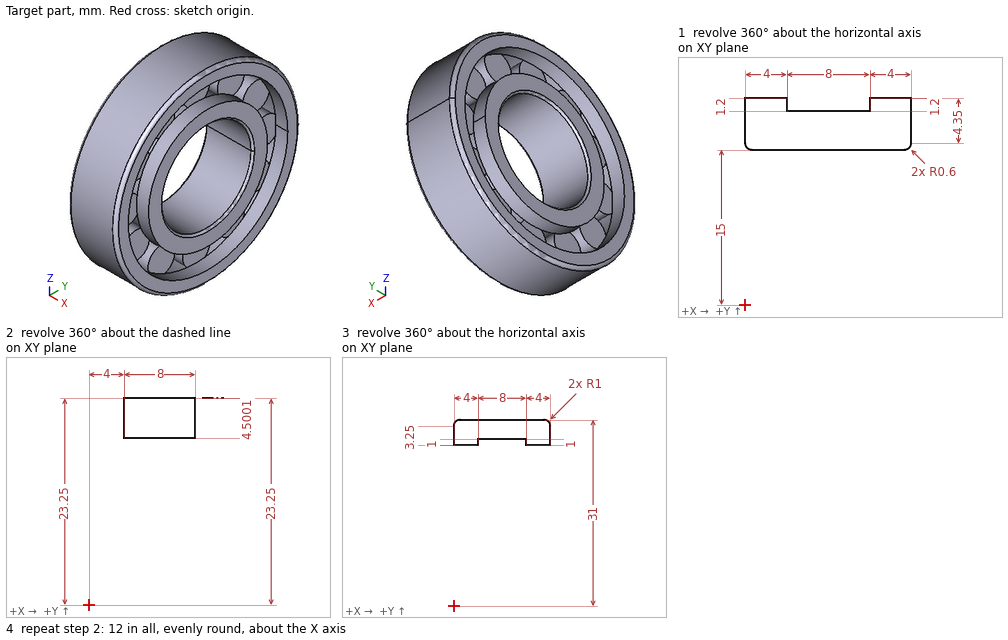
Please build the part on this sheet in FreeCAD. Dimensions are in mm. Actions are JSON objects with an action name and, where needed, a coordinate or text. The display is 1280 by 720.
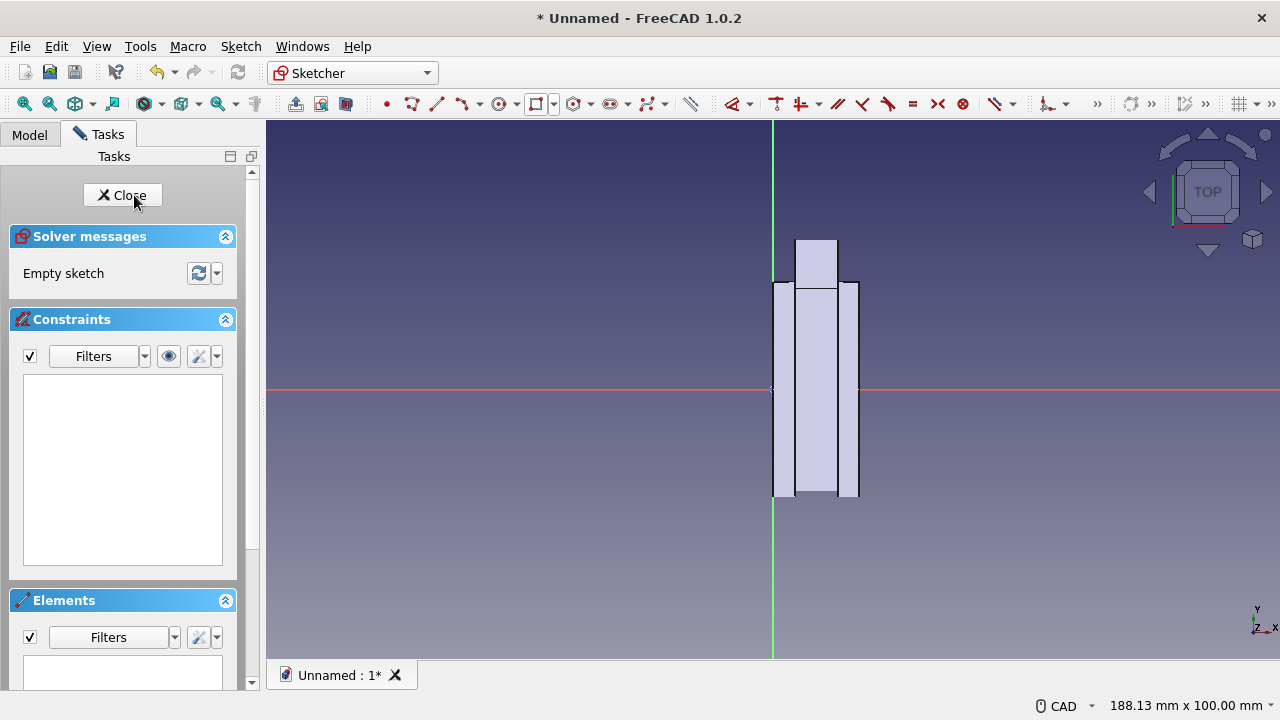
{"action": "left_click", "coordinate": [346, 104]}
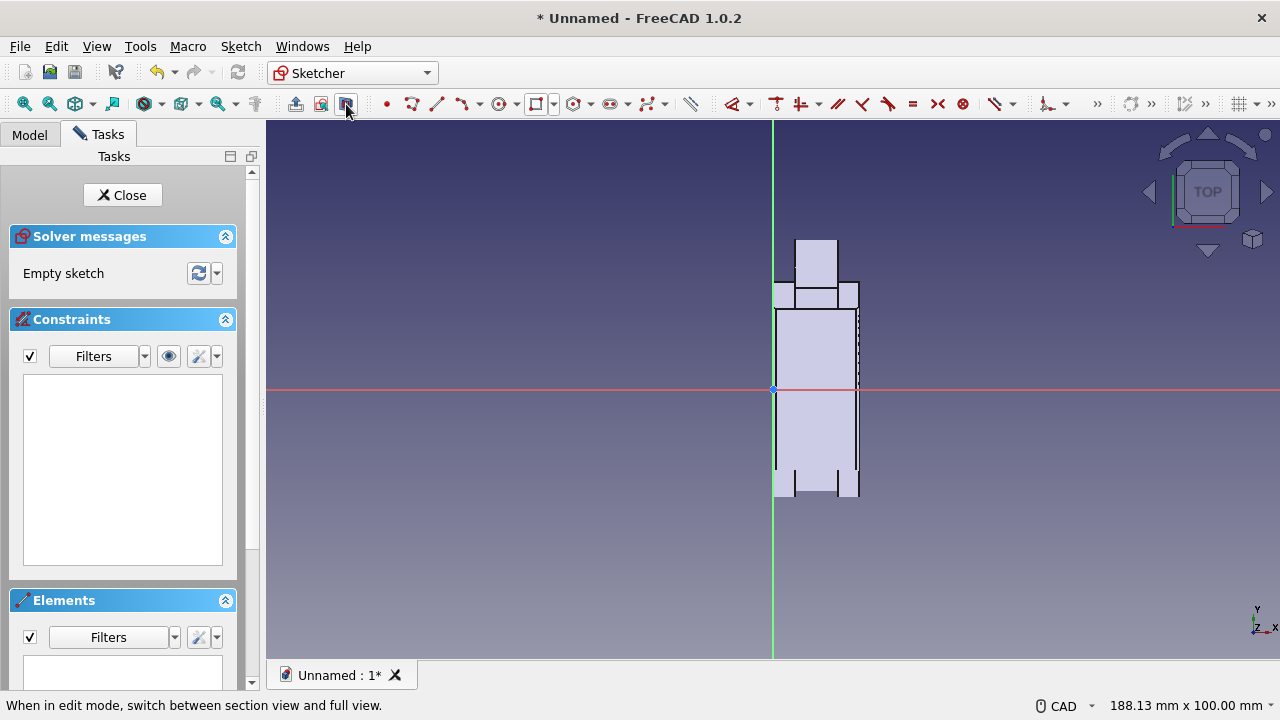
{"action": "scroll", "coordinate": [907, 238], "scroll_direction": "up", "scroll_amount": 4}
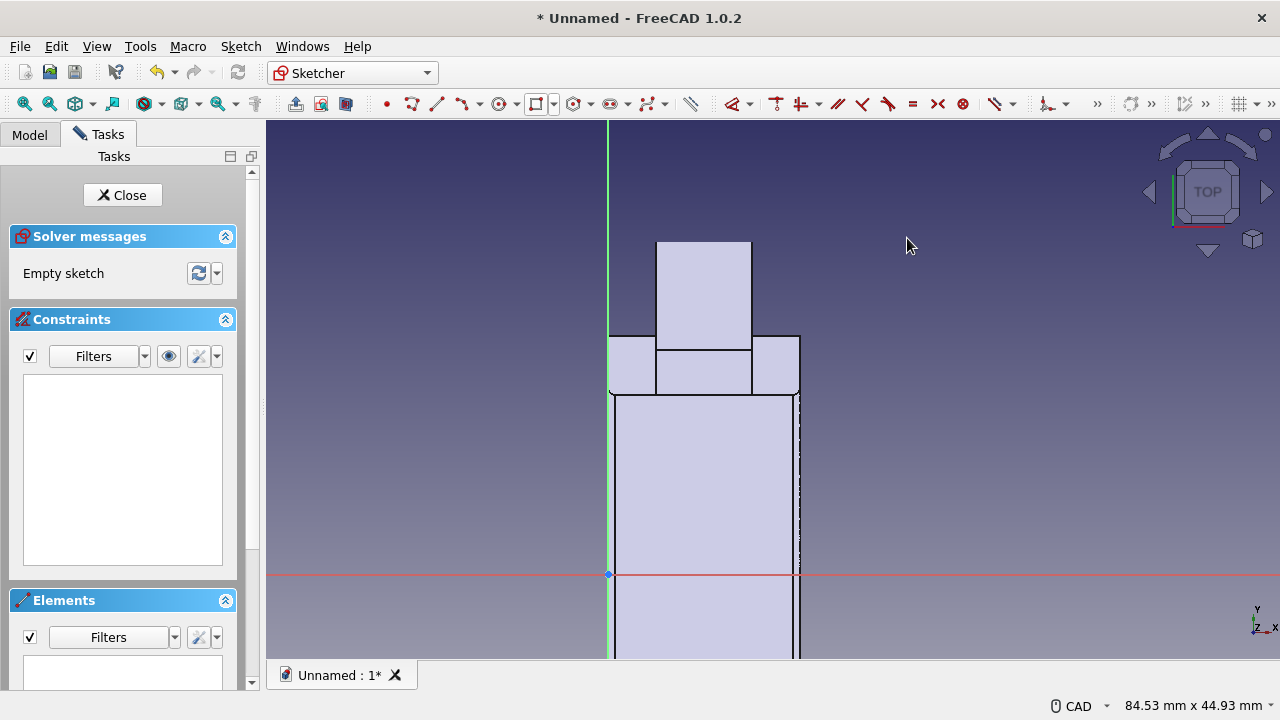
{"action": "left_click", "coordinate": [437, 104]}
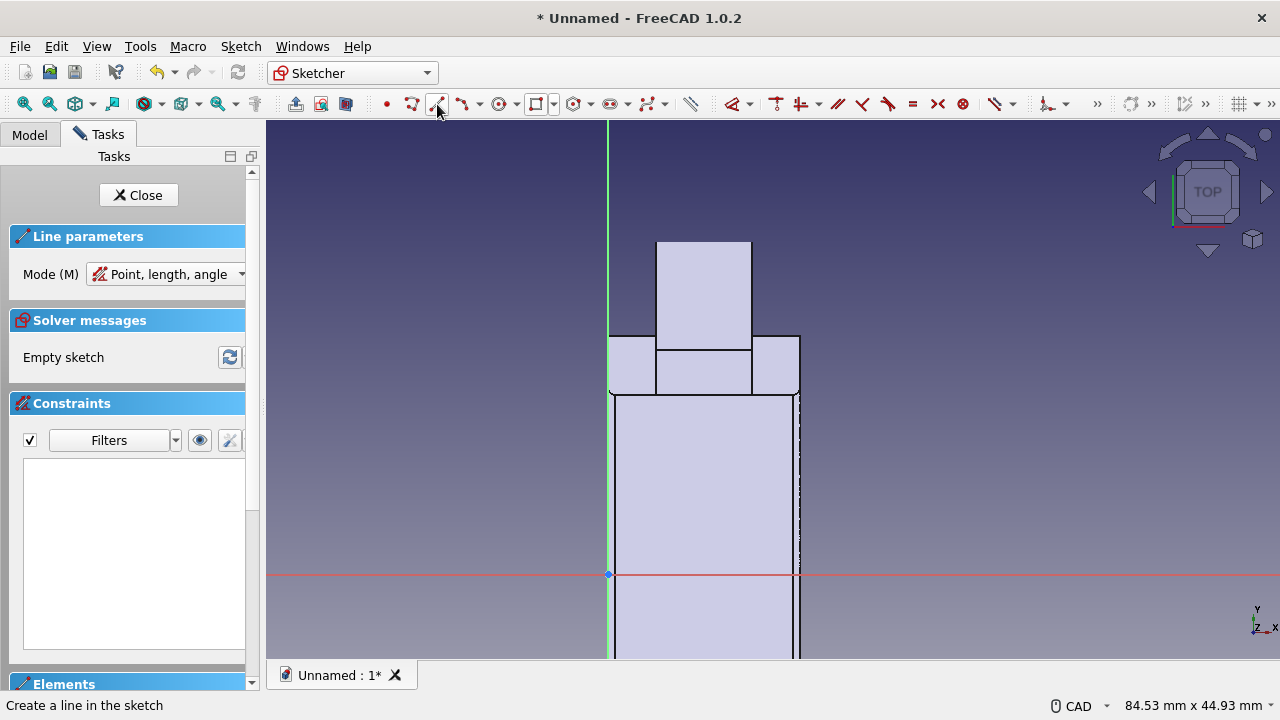
{"action": "left_click", "coordinate": [788, 203]}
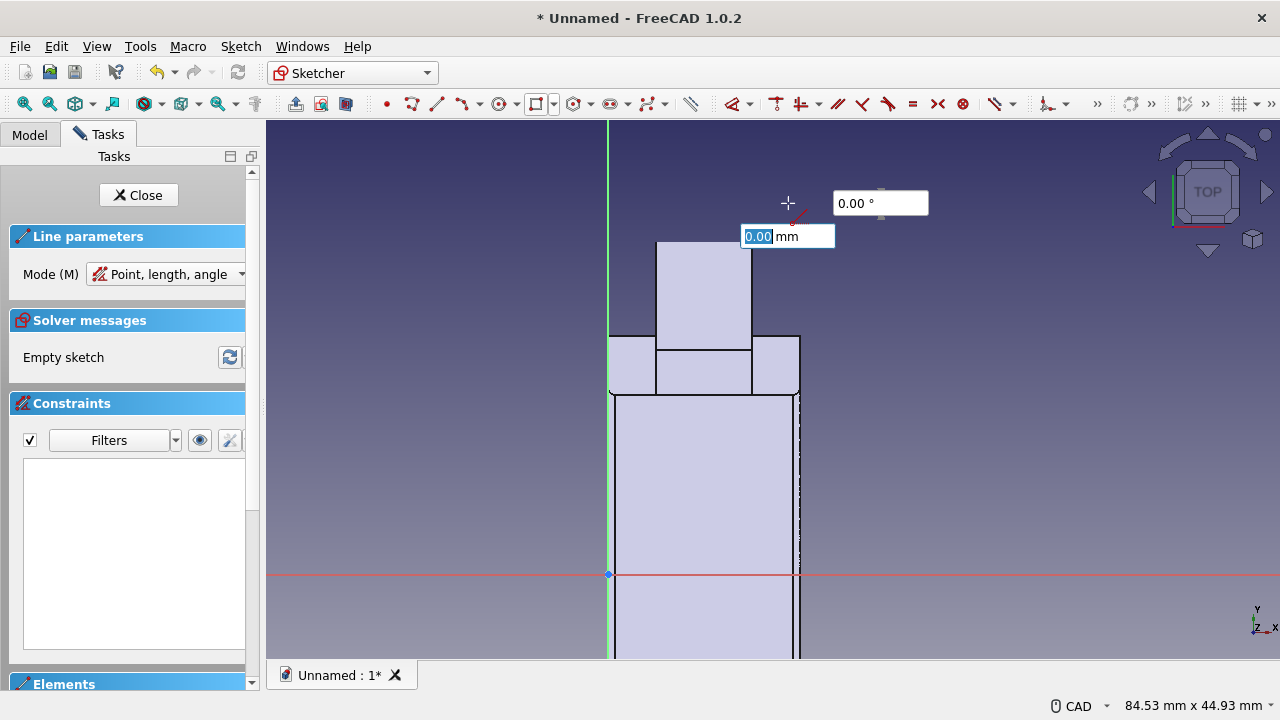
{"action": "scroll", "coordinate": [620, 203], "scroll_direction": "up", "scroll_amount": 2}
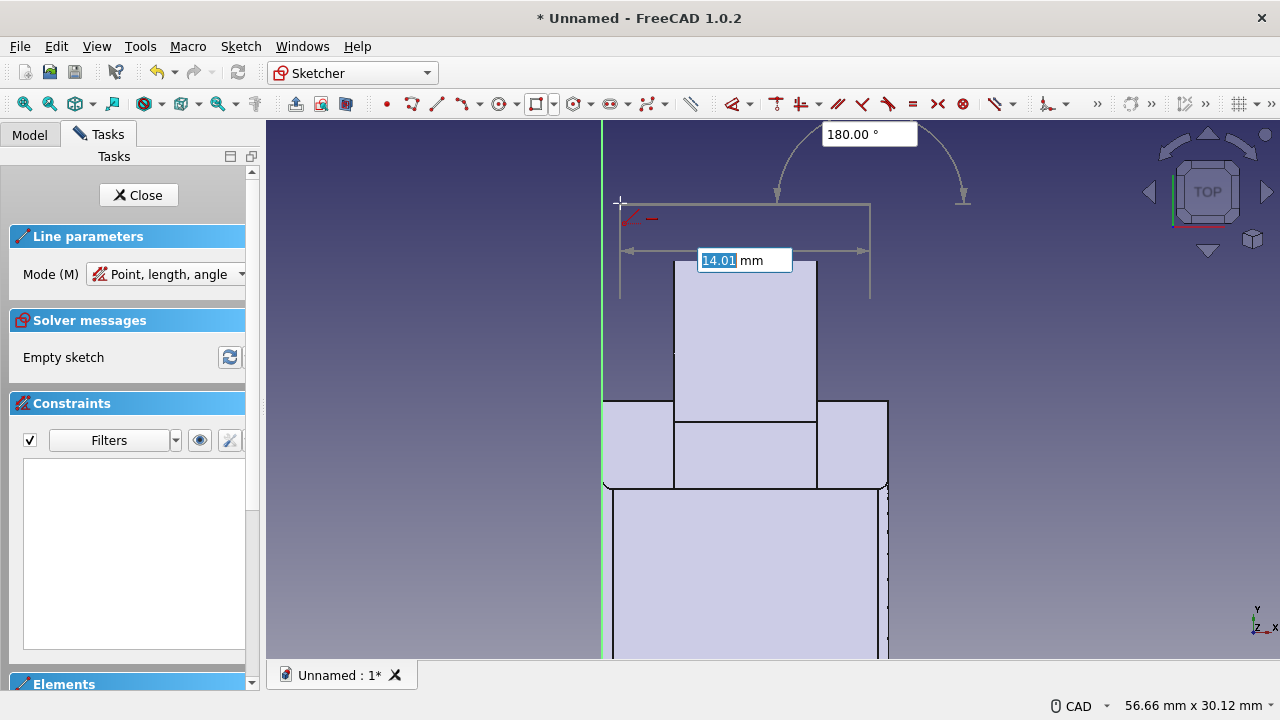
{"action": "left_click", "coordinate": [620, 203]}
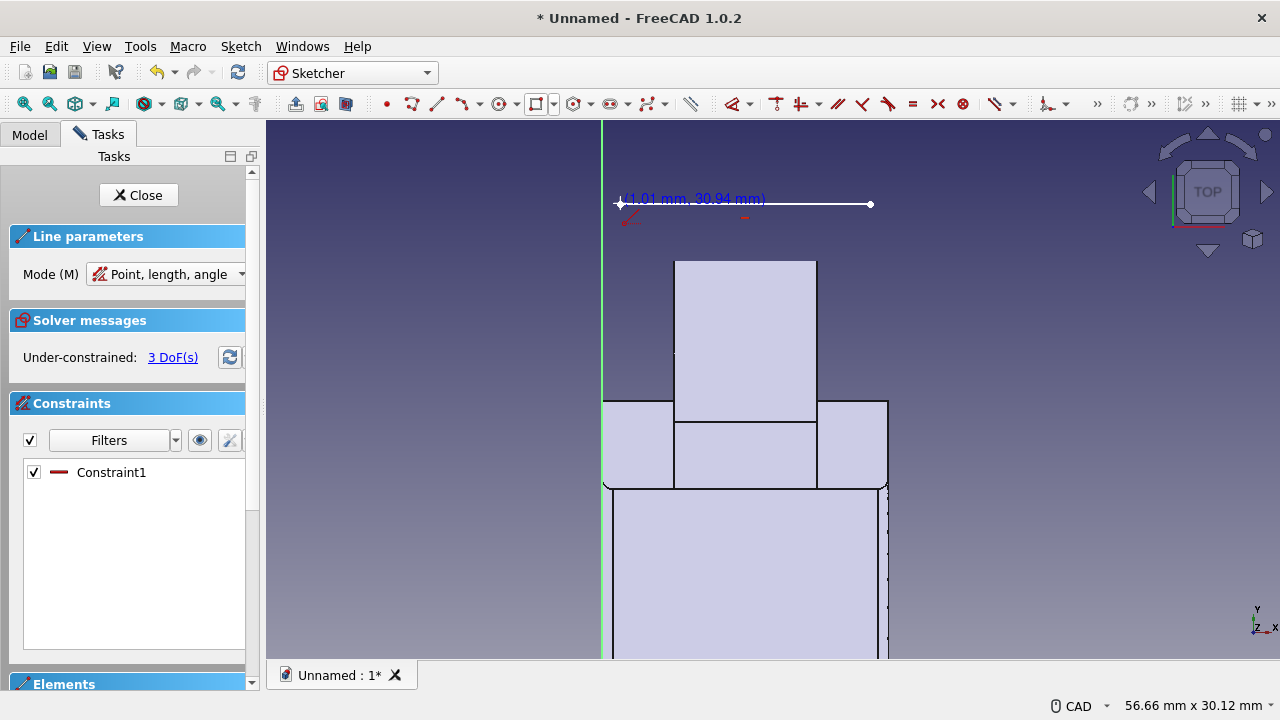
{"action": "left_click", "coordinate": [412, 104]}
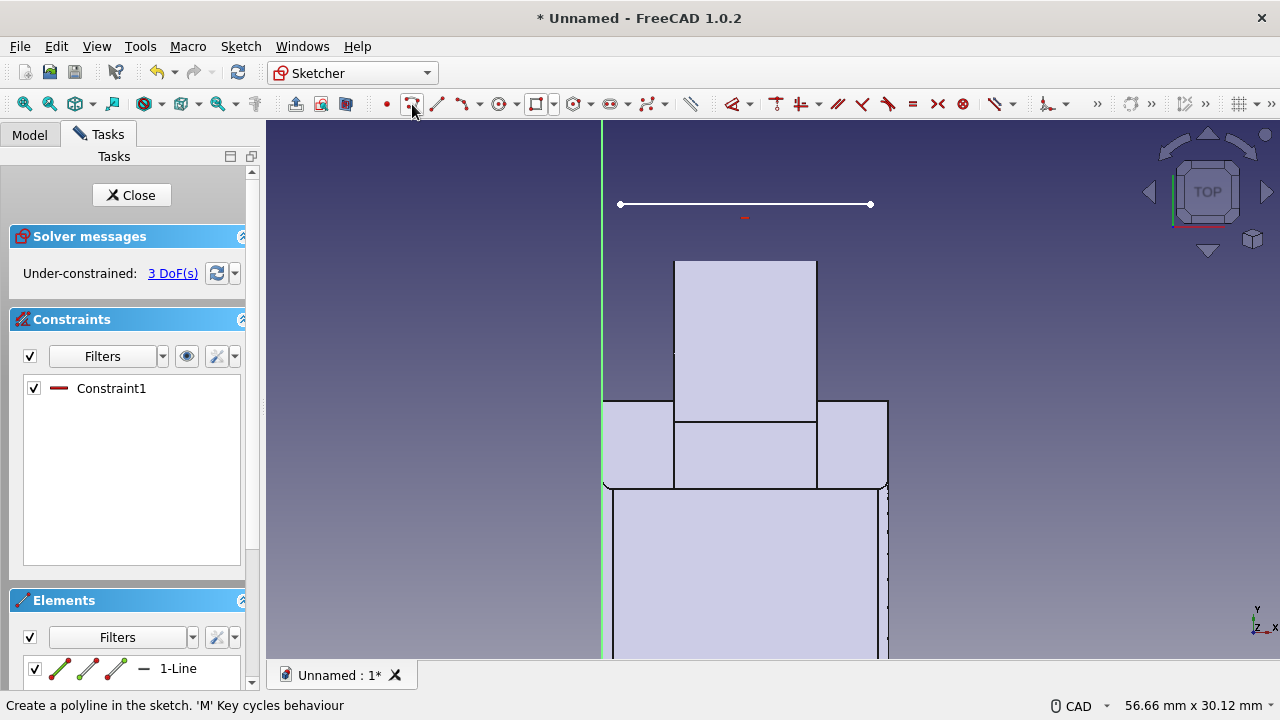
{"action": "left_click", "coordinate": [602, 221]}
{"action": "left_click", "coordinate": [611, 279]}
{"action": "left_click", "coordinate": [674, 279]}
{"action": "left_click", "coordinate": [674, 261]}
{"action": "left_click", "coordinate": [817, 261]}
{"action": "left_click", "coordinate": [817, 279]}
{"action": "left_click", "coordinate": [888, 279]}
{"action": "left_click", "coordinate": [888, 221]}
{"action": "right_click", "coordinate": [888, 221]}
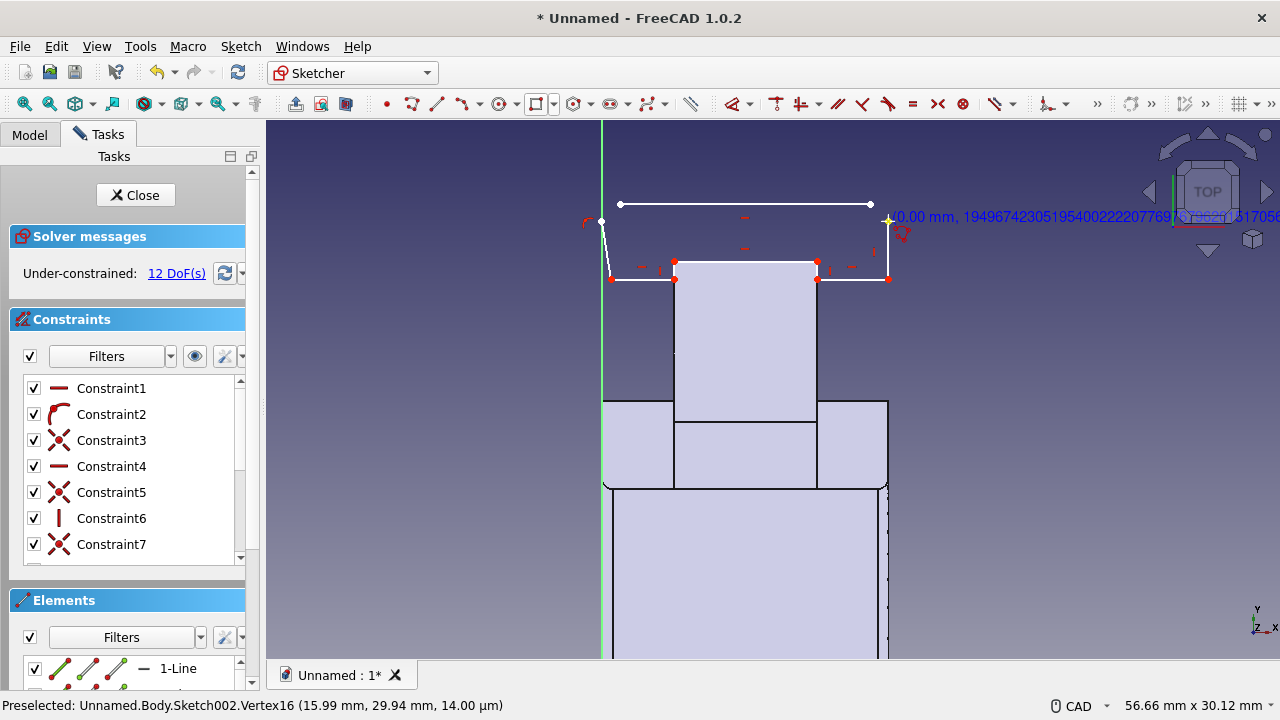
{"action": "left_click", "coordinate": [462, 104]}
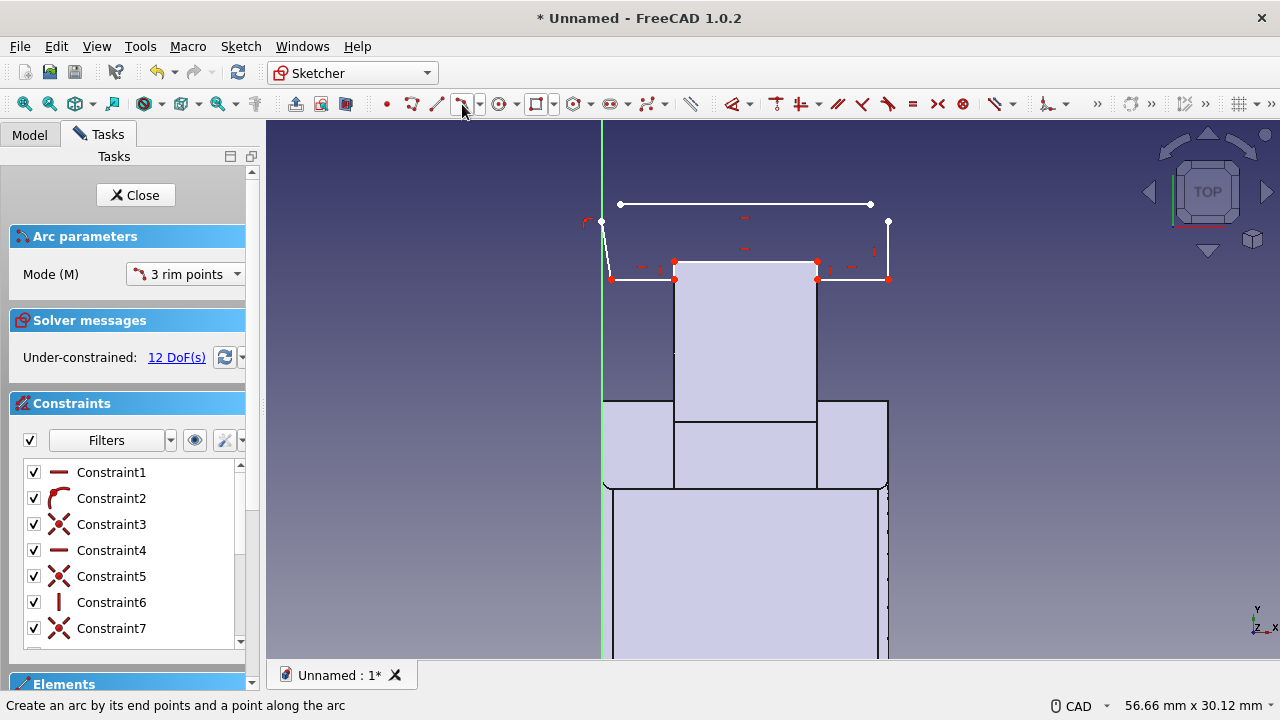
{"action": "left_click", "coordinate": [620, 204]}
{"action": "left_click", "coordinate": [602, 222]}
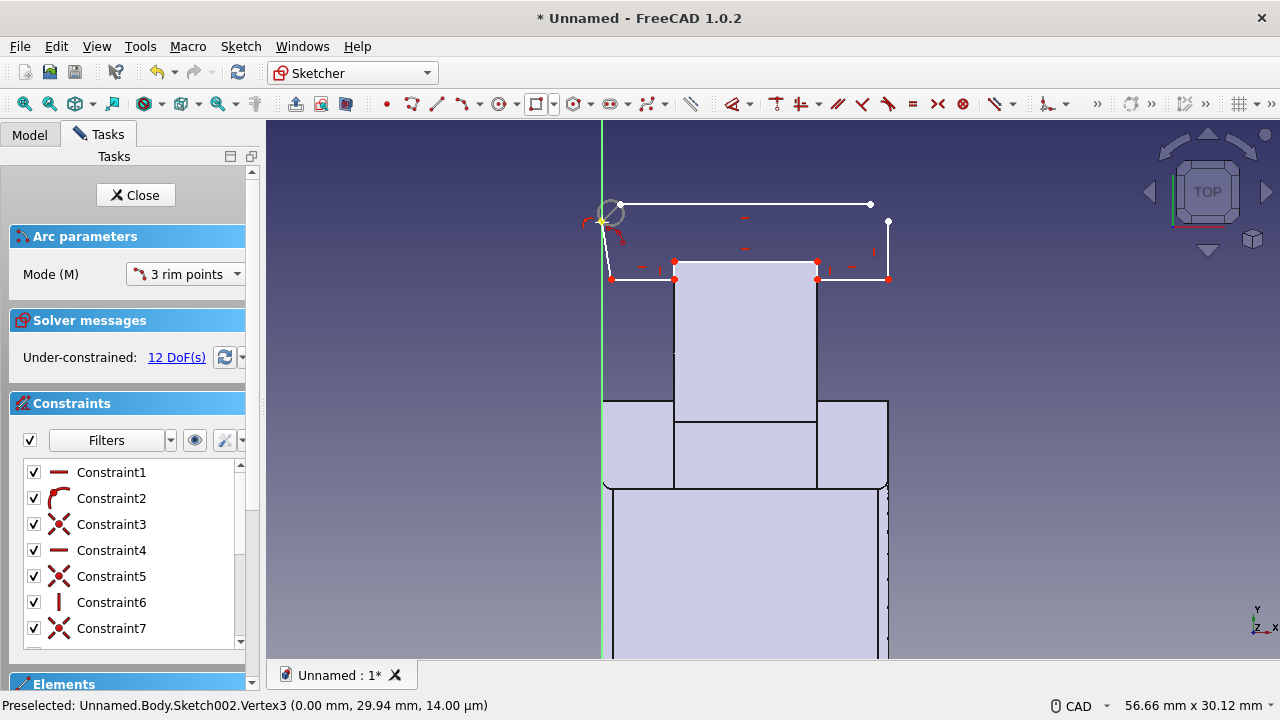
{"action": "scroll", "coordinate": [607, 208], "scroll_direction": "up", "scroll_amount": 6}